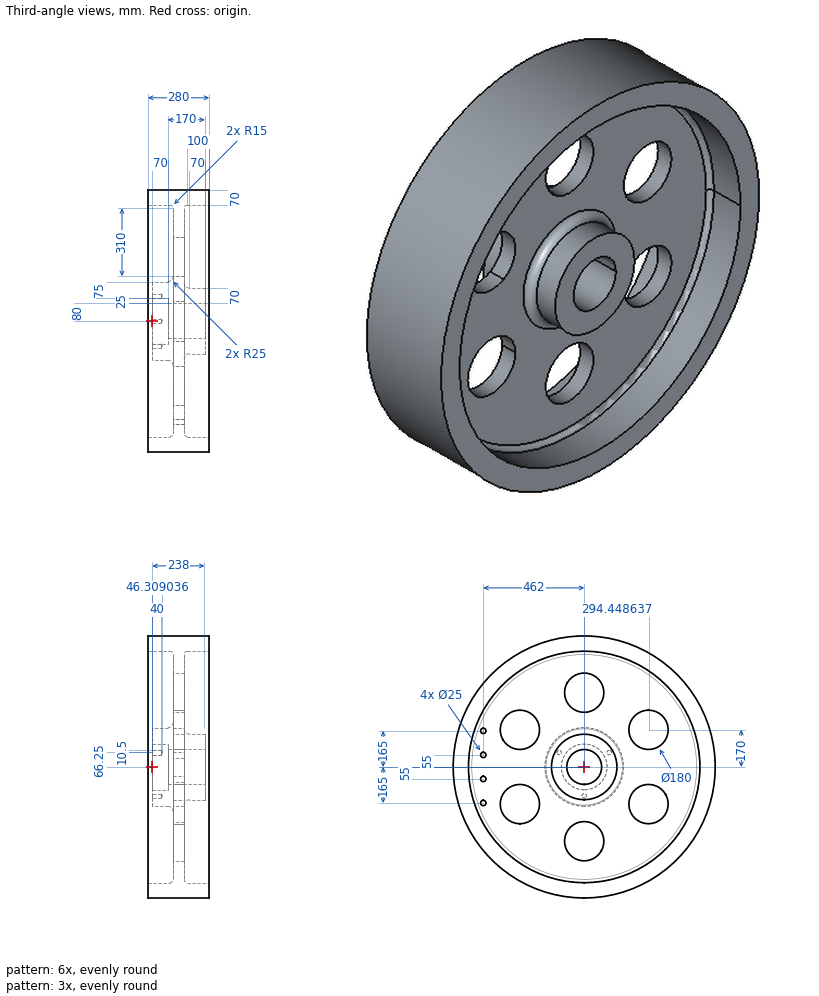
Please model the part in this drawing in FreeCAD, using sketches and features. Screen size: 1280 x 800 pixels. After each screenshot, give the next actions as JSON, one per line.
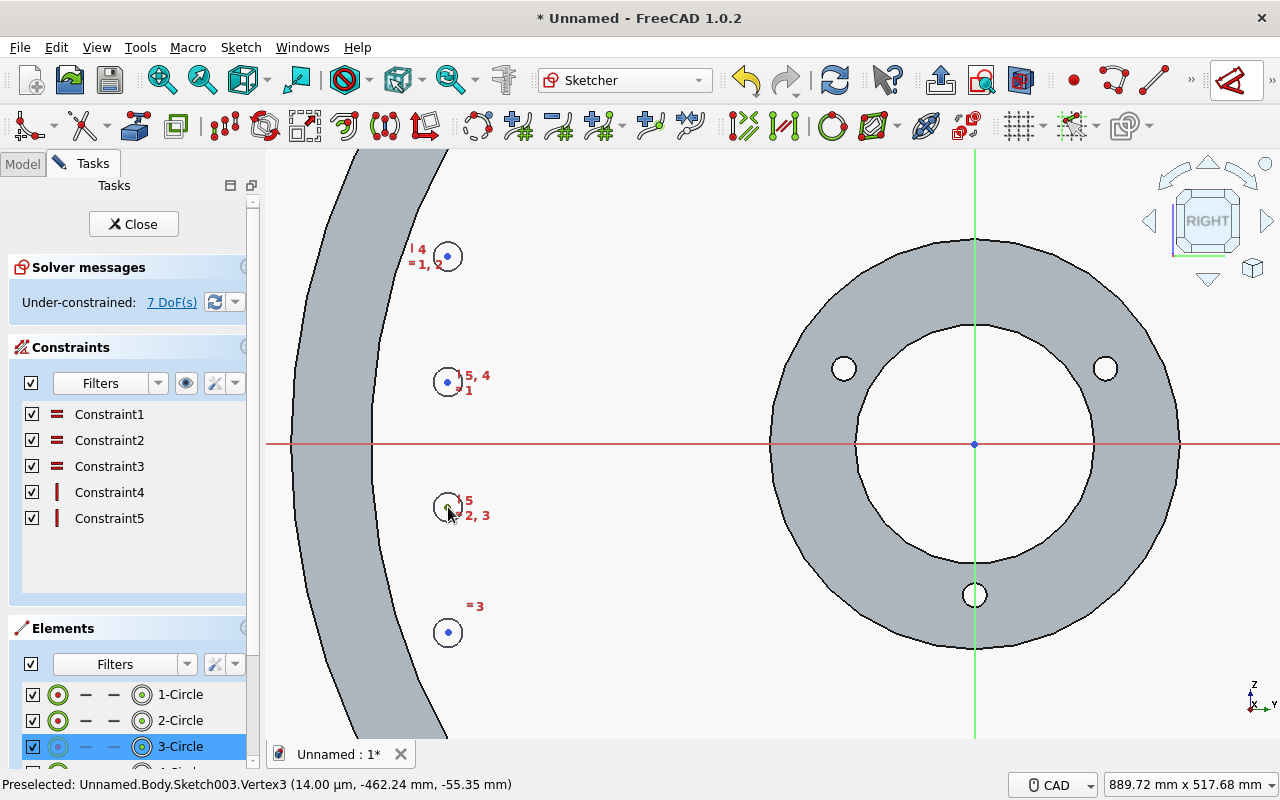
{"action": "left_click", "coordinate": [448, 633]}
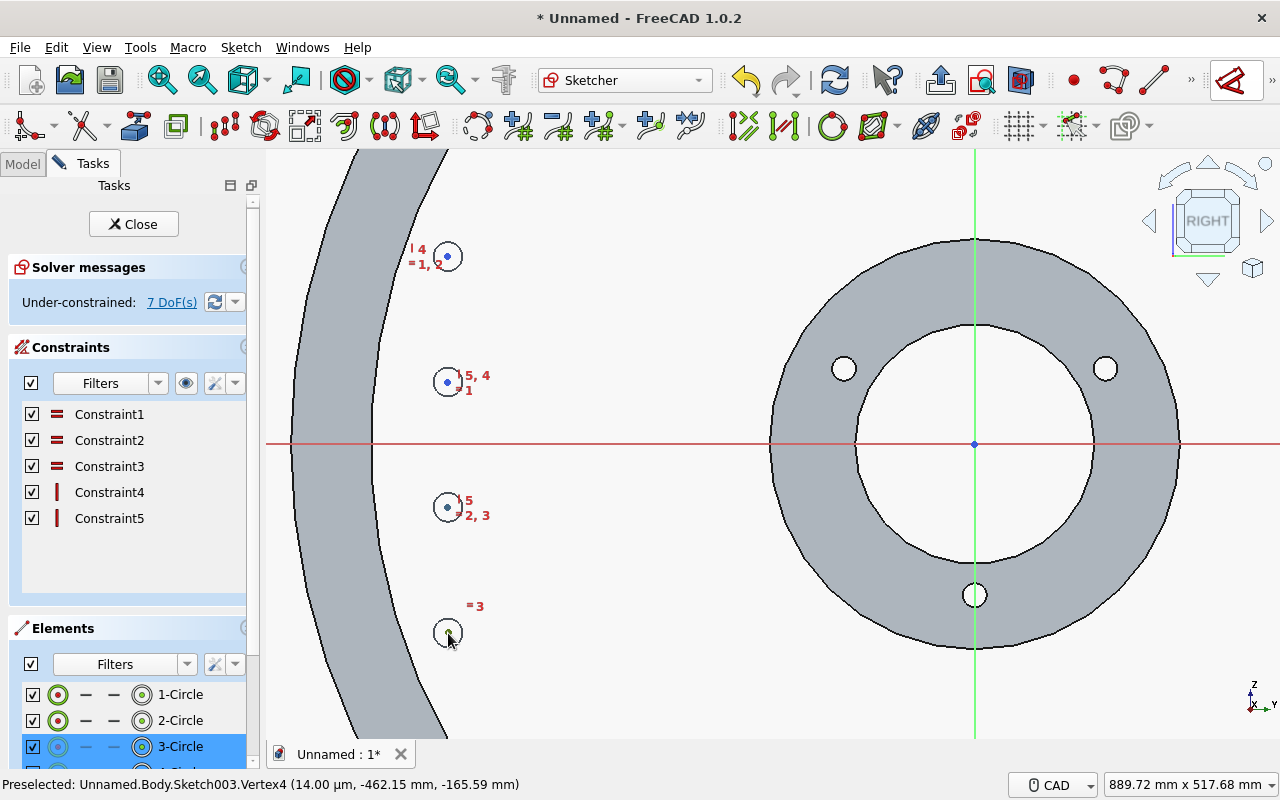
{"action": "key", "text": "v"}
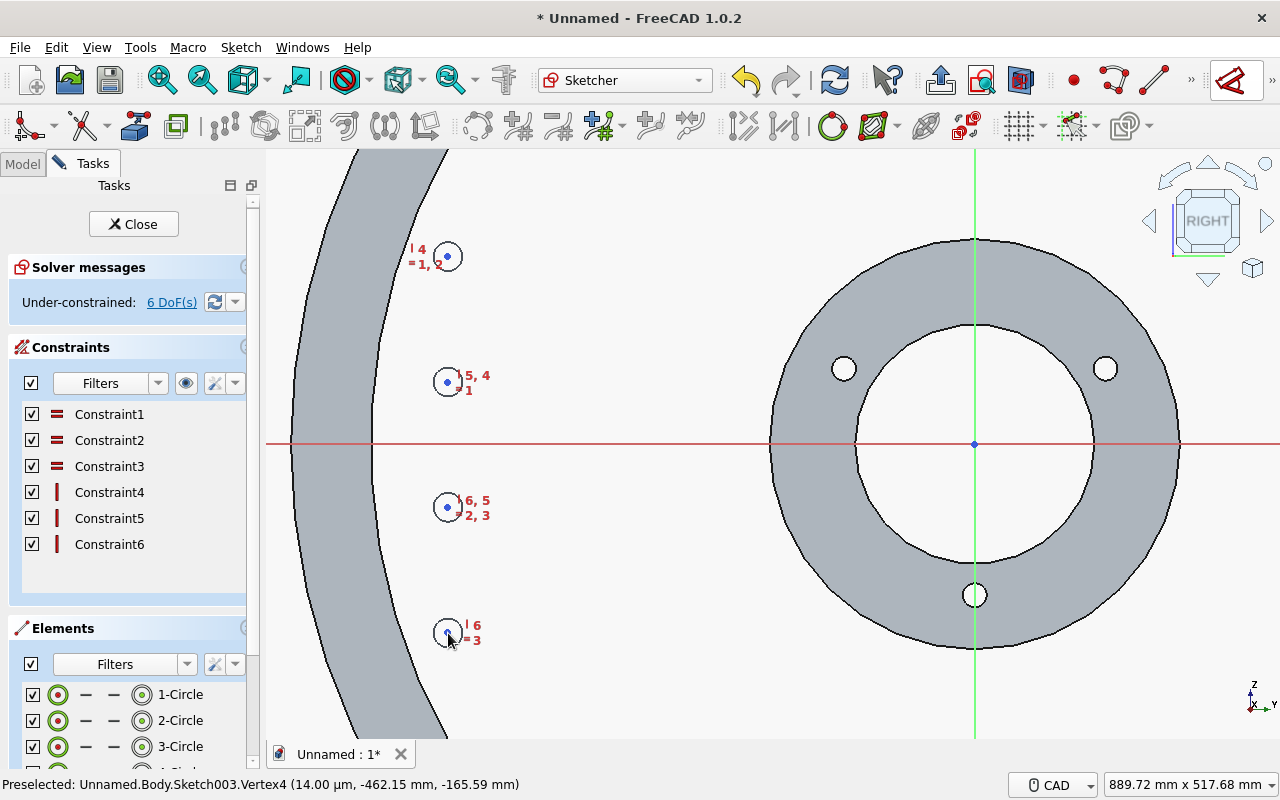
{"action": "scroll", "coordinate": [458, 372], "scroll_direction": "up", "scroll_amount": 2}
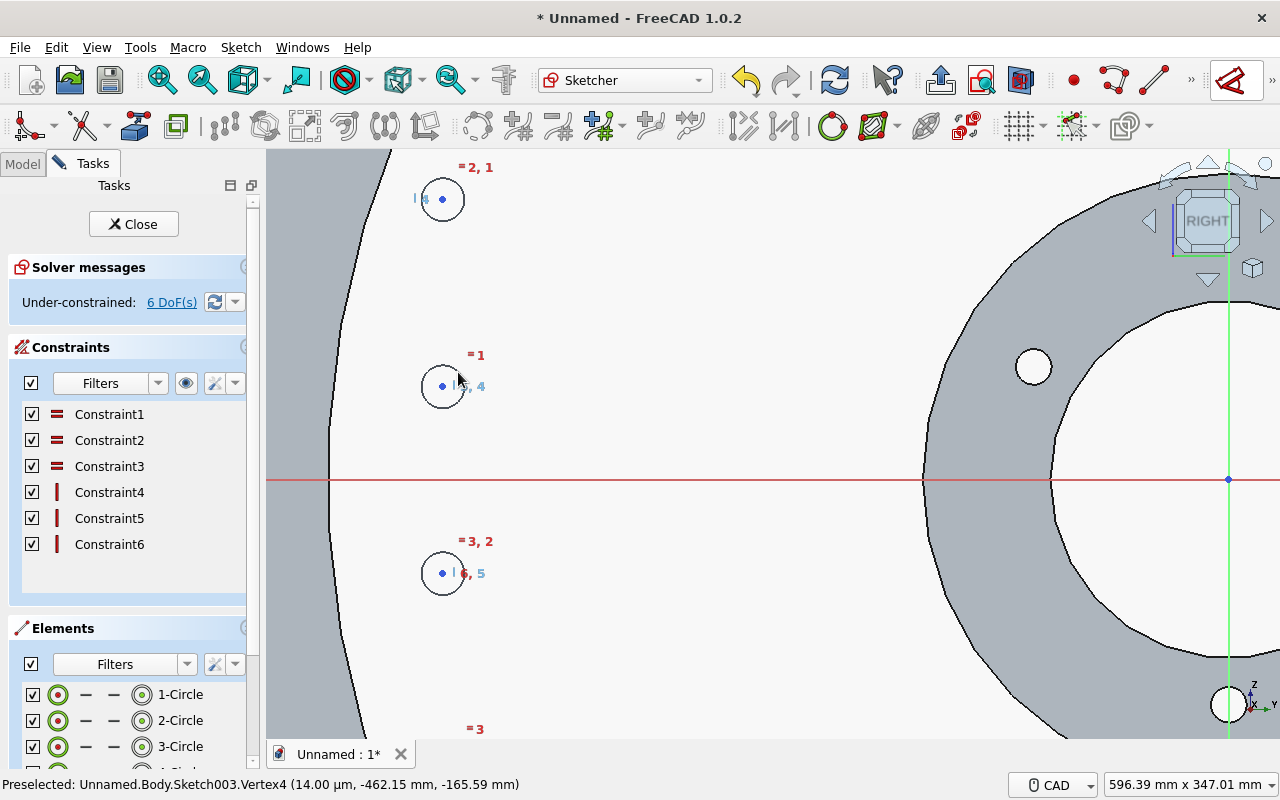
{"action": "left_click", "coordinate": [458, 372]}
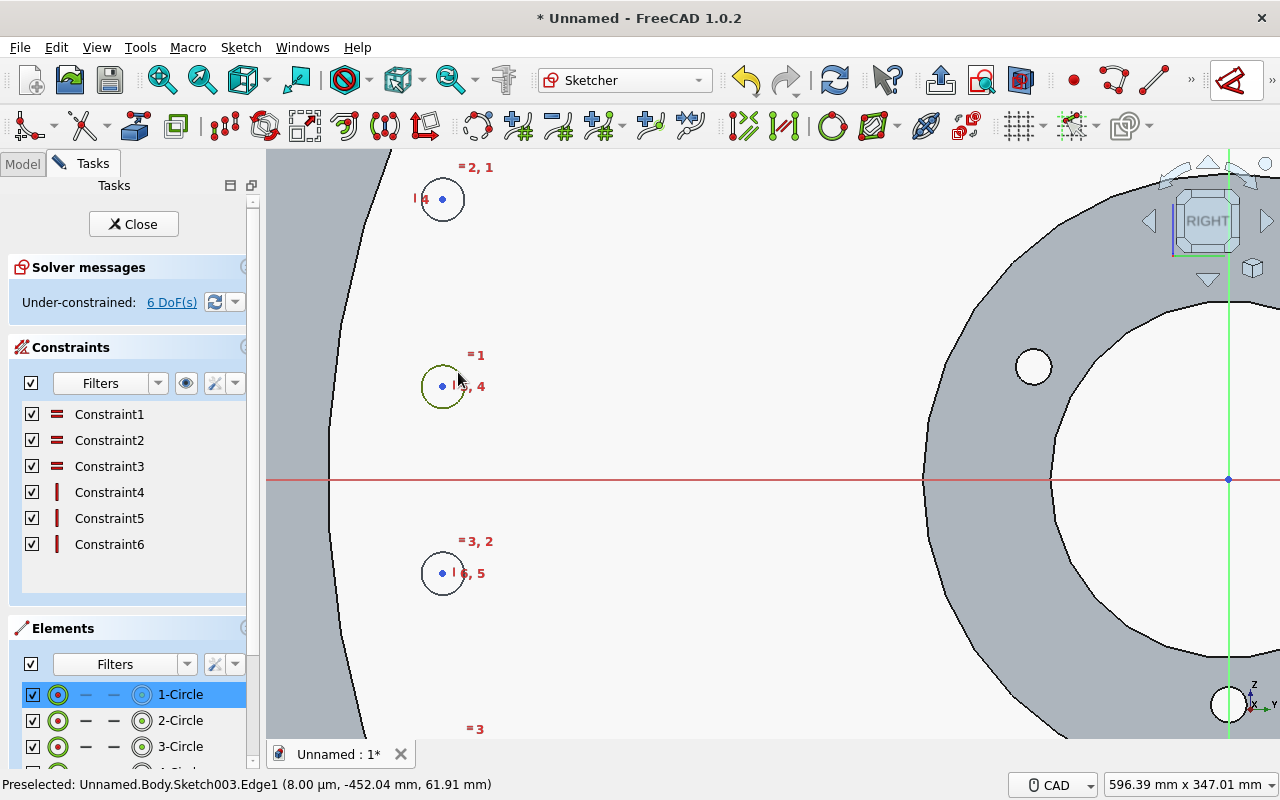
{"action": "key", "text": "k o"}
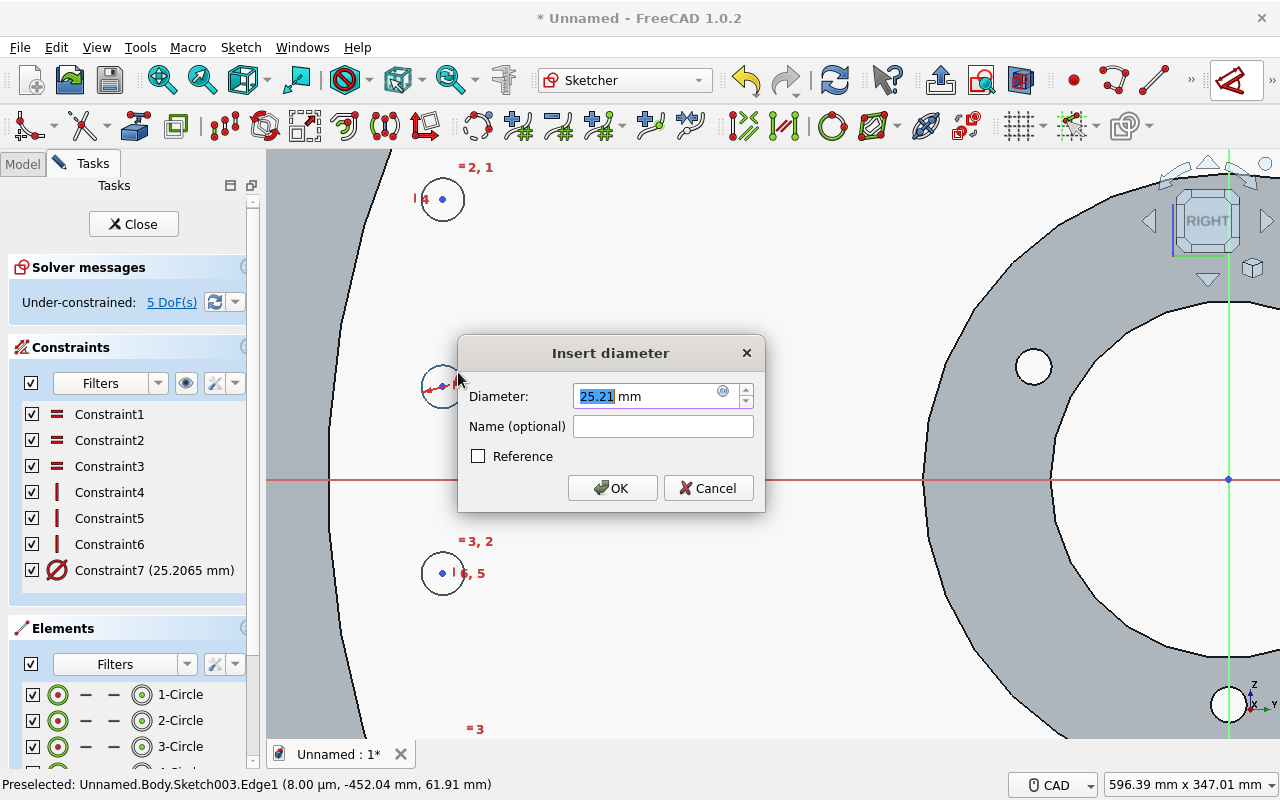
{"action": "type", "text": "25"}
{"action": "key", "text": "Return"}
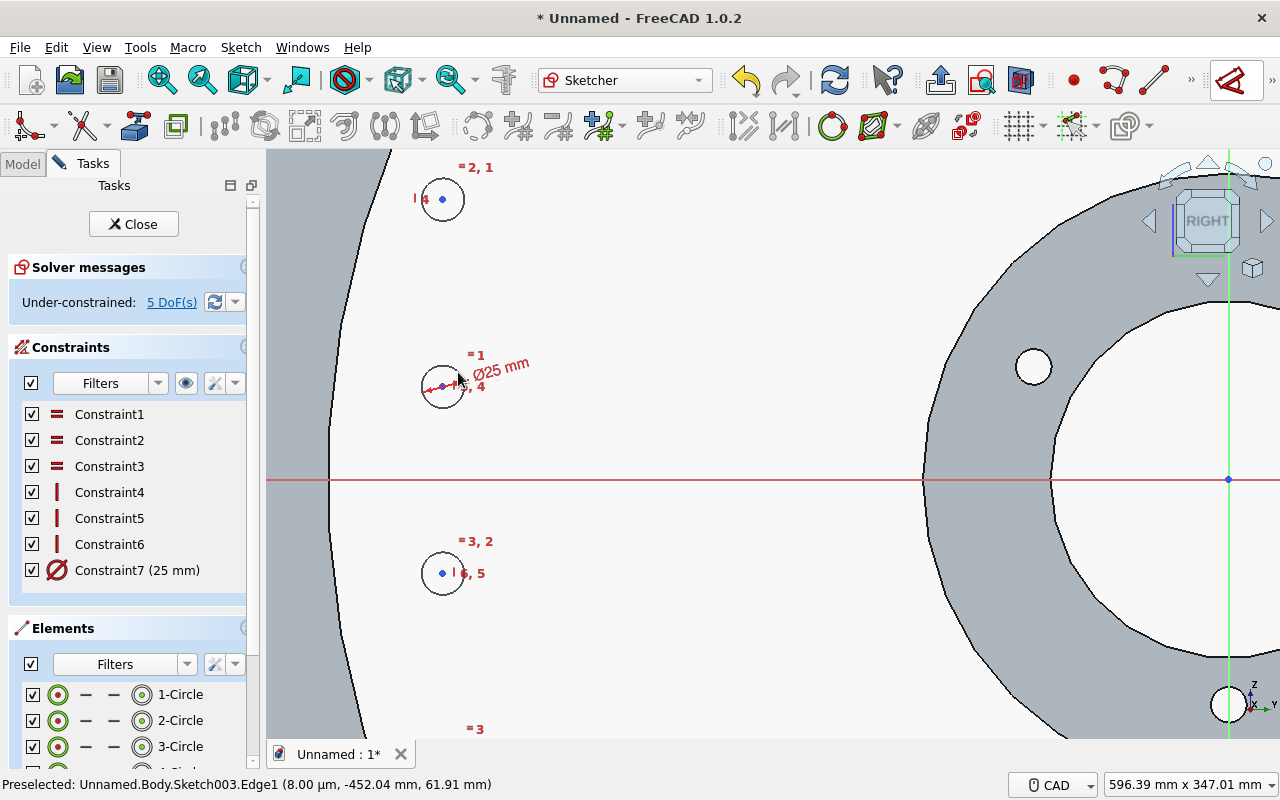
{"action": "left_click", "coordinate": [443, 387]}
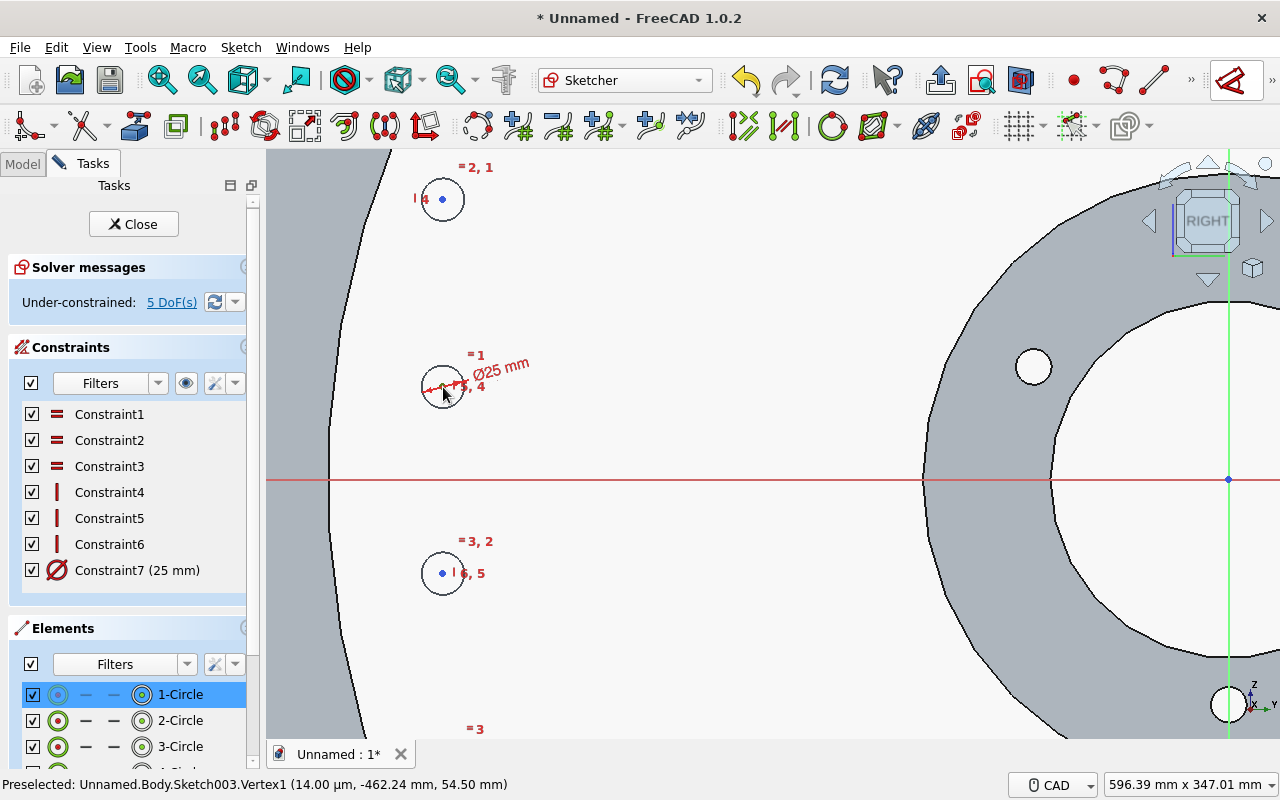
{"action": "left_click", "coordinate": [1258, 80]}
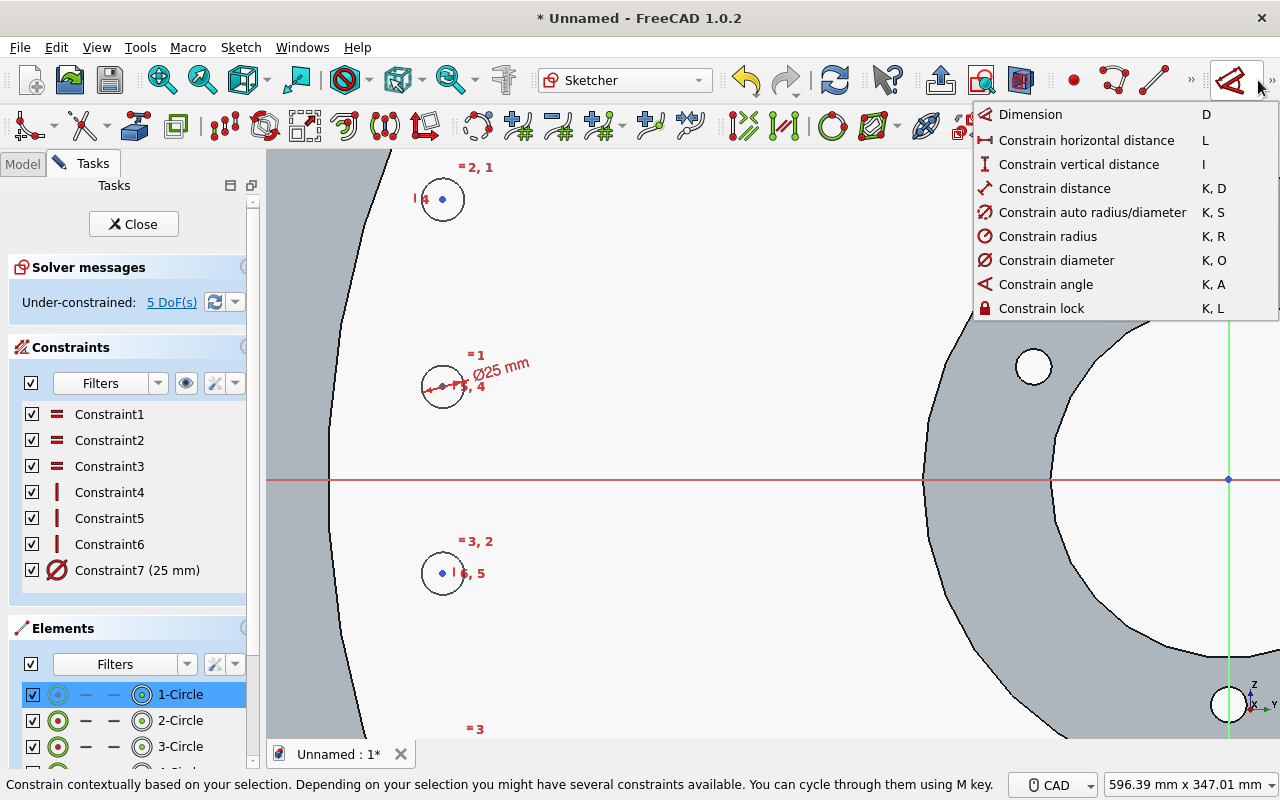
{"action": "left_click", "coordinate": [1126, 164]}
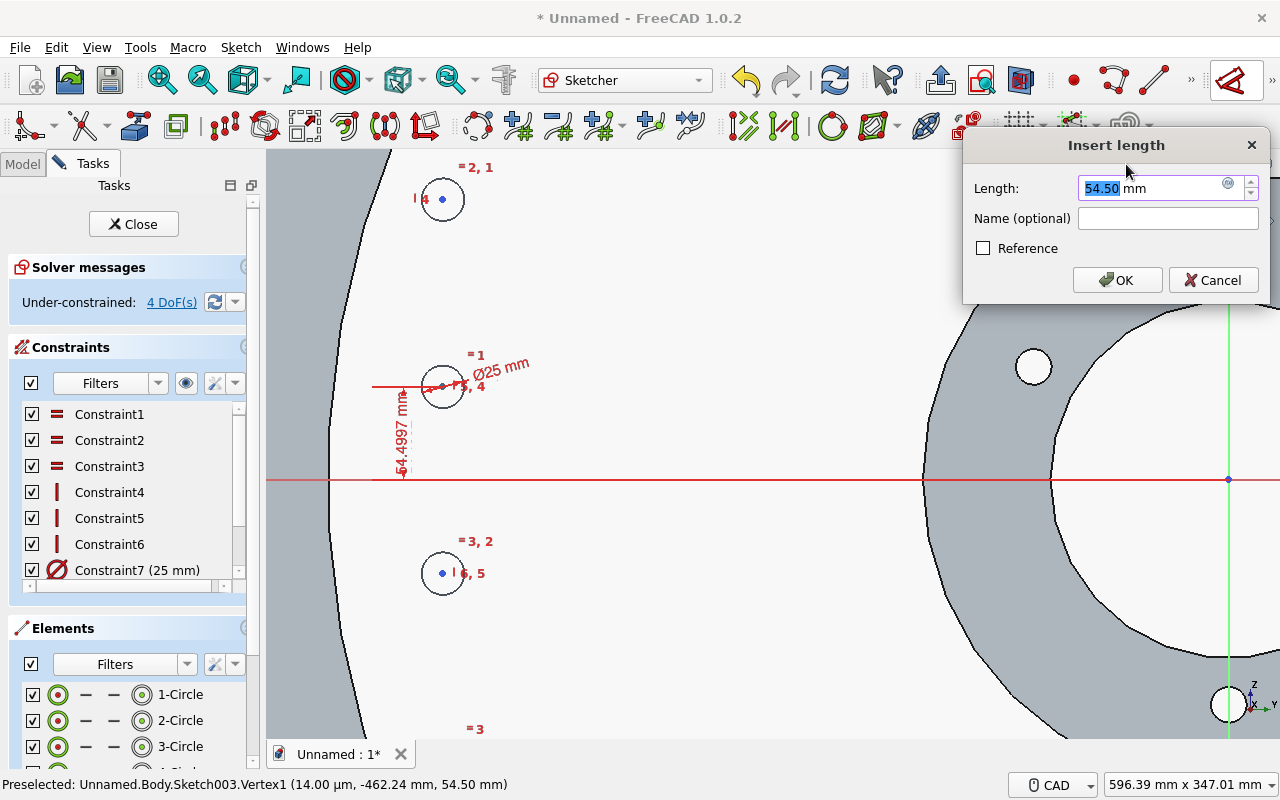
{"action": "type", "text": "55"}
{"action": "key", "text": "Return"}